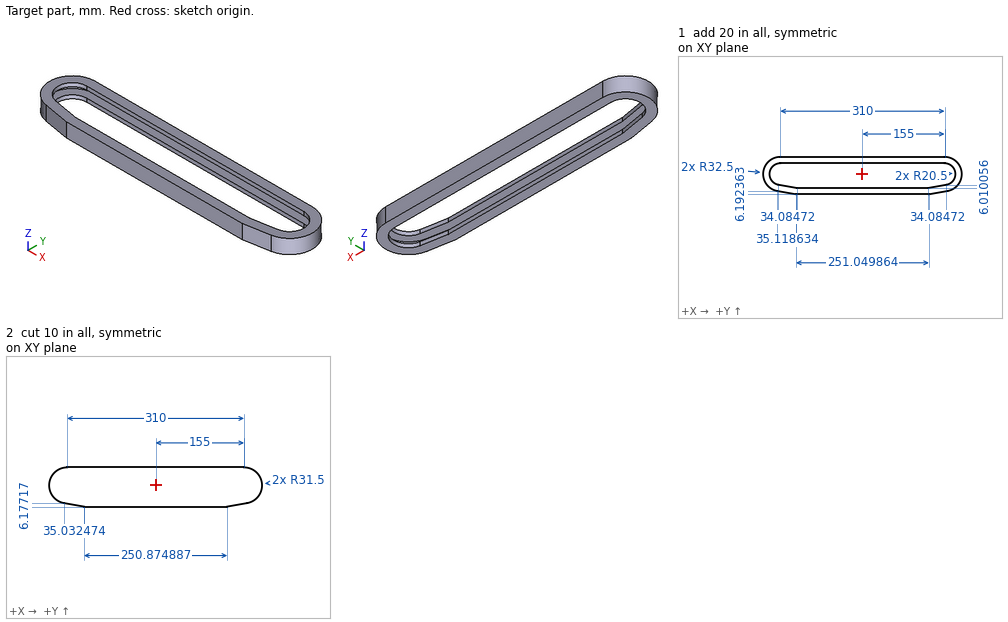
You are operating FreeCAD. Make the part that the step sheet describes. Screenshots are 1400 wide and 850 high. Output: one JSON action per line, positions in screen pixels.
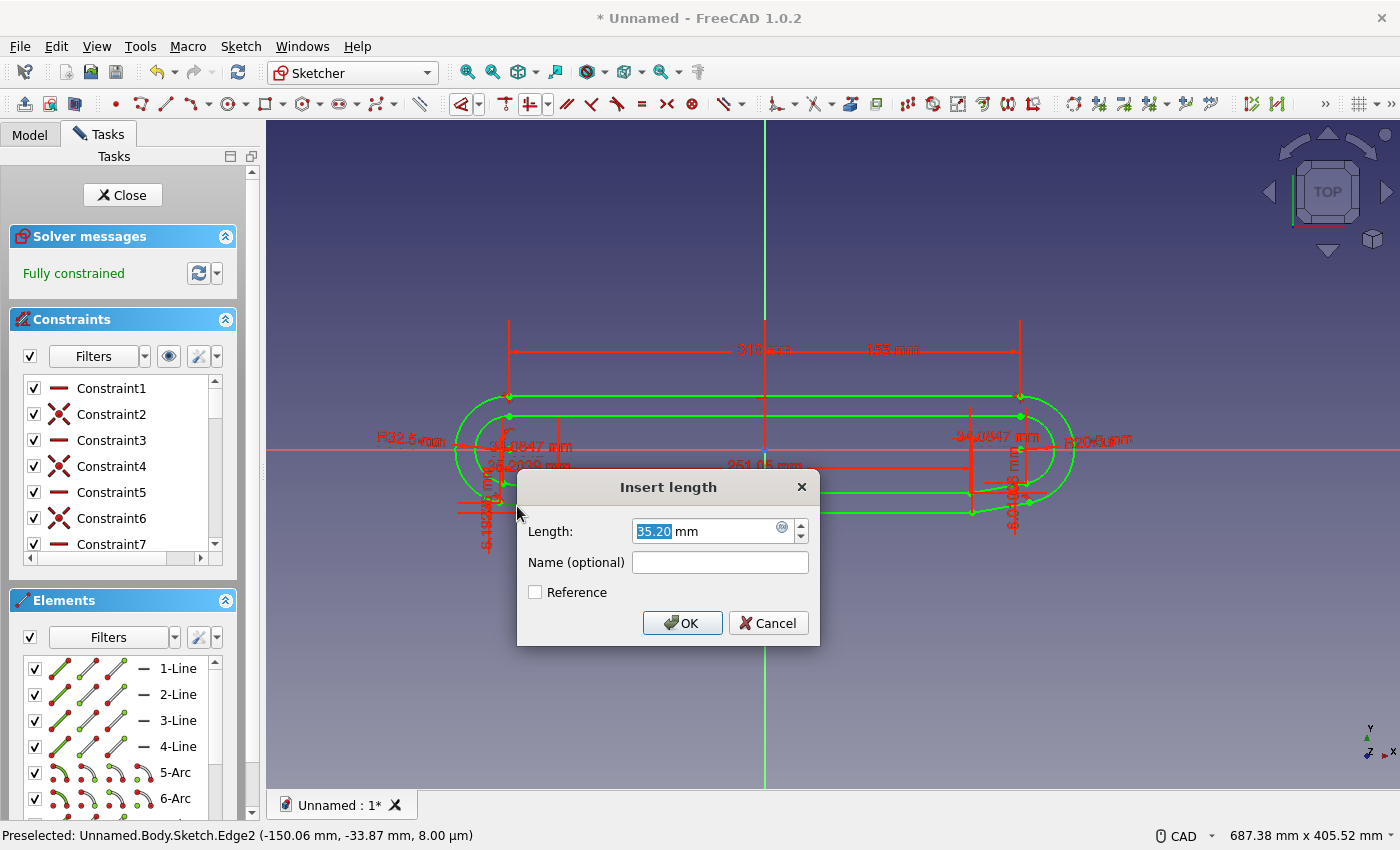
{"action": "type", "text": "35.118634"}
{"action": "key", "text": "Return"}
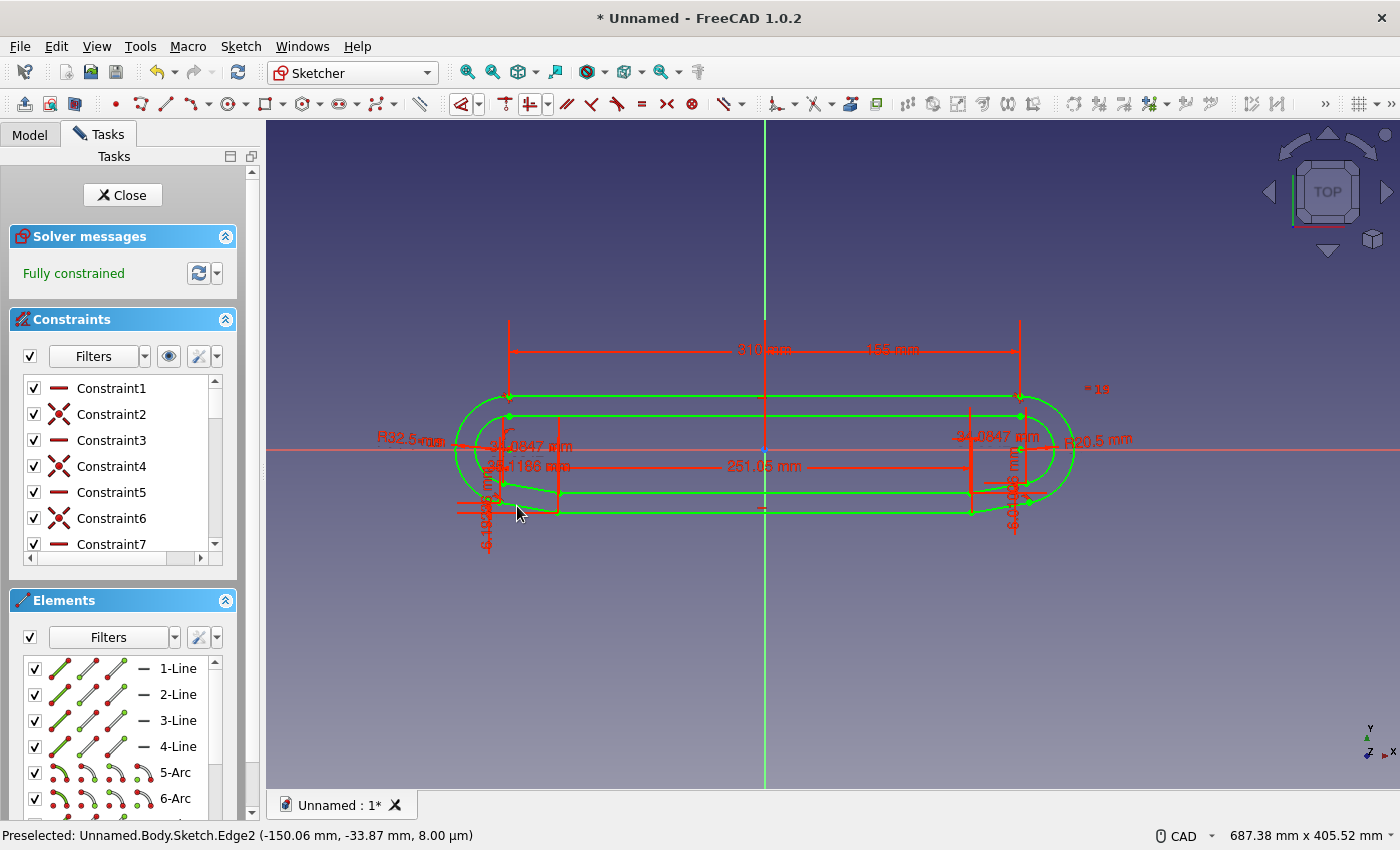
{"action": "left_click", "coordinate": [123, 195]}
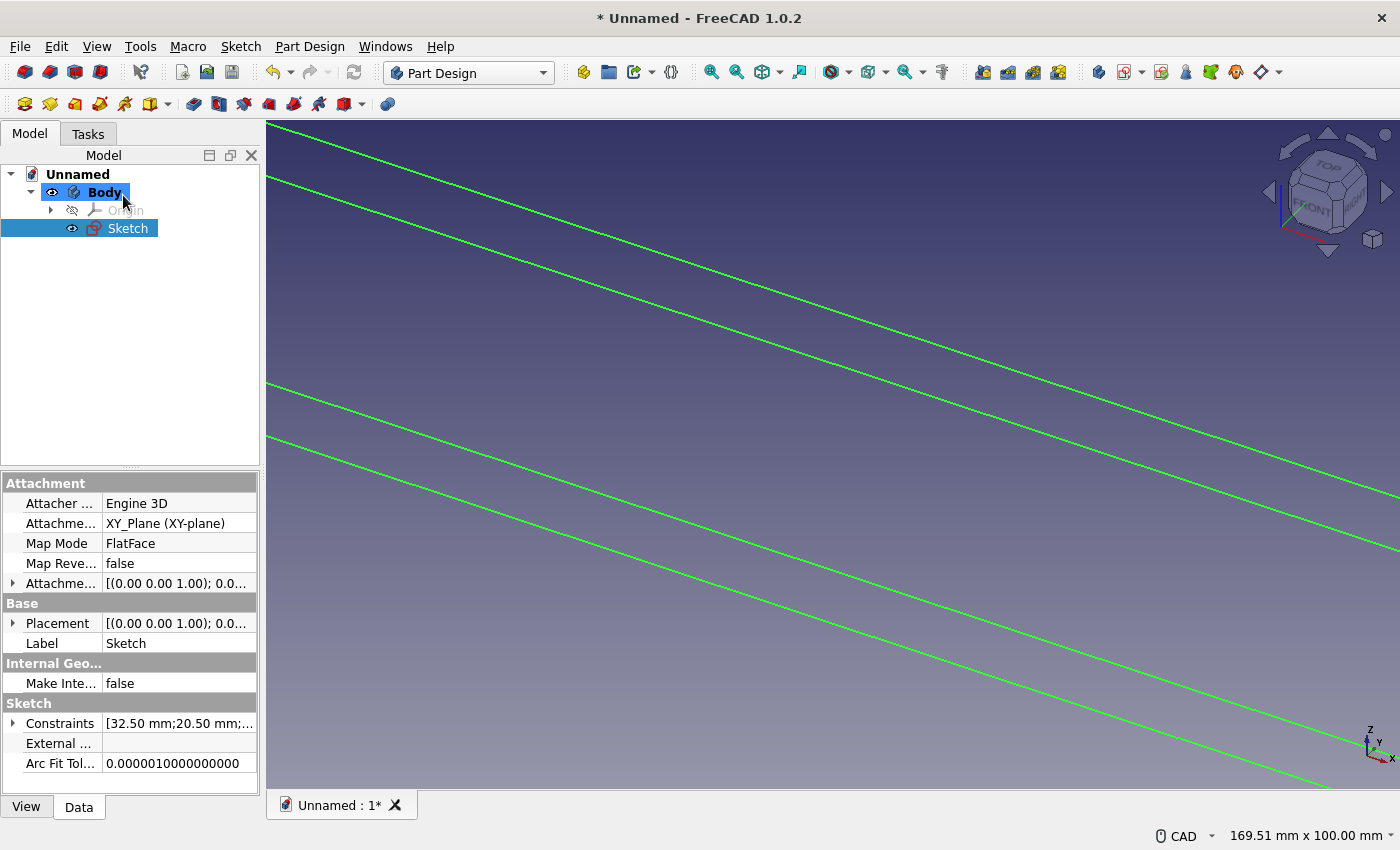
{"action": "left_click", "coordinate": [25, 104]}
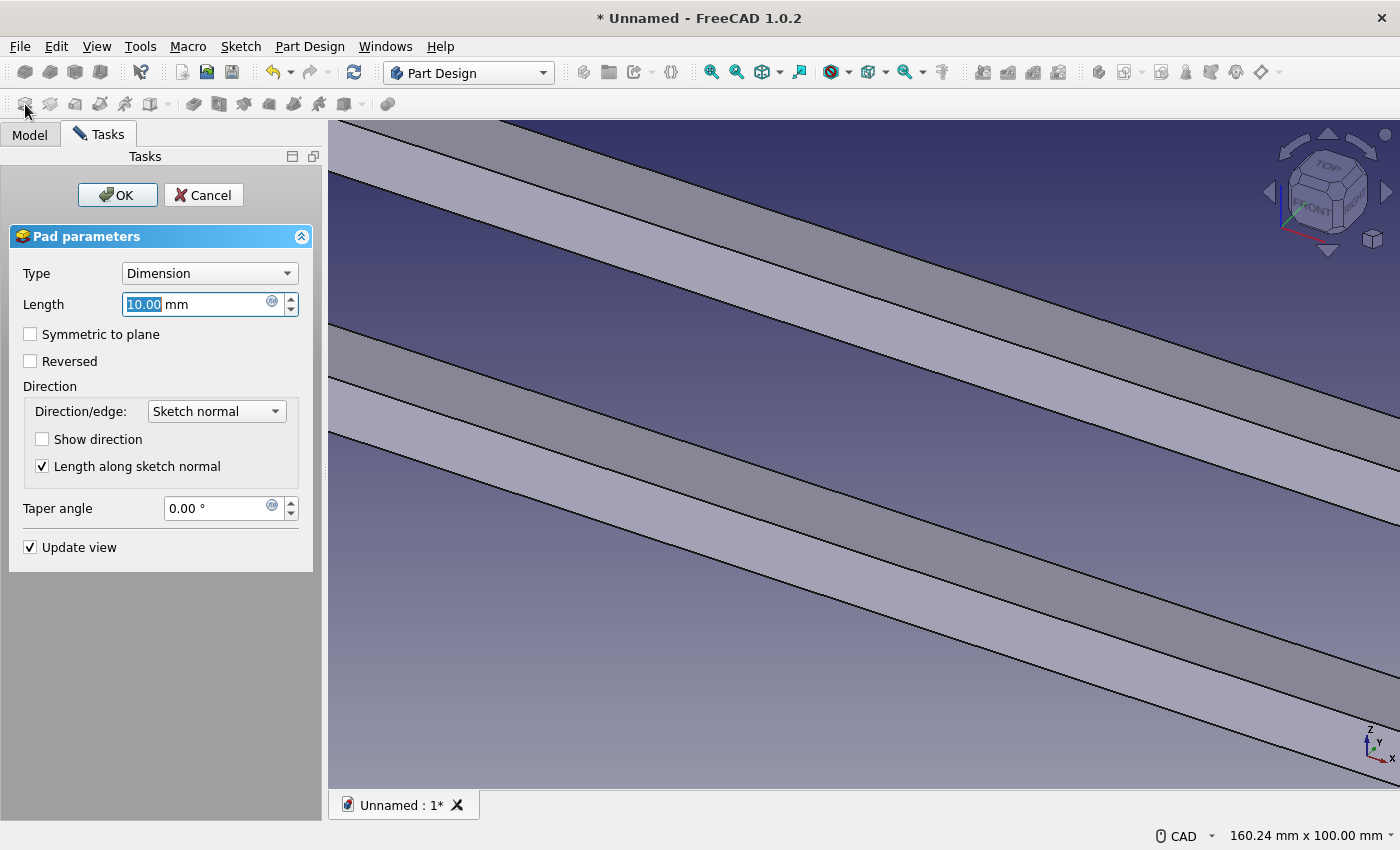
{"action": "type", "text": "20"}
{"action": "key", "text": "Tab"}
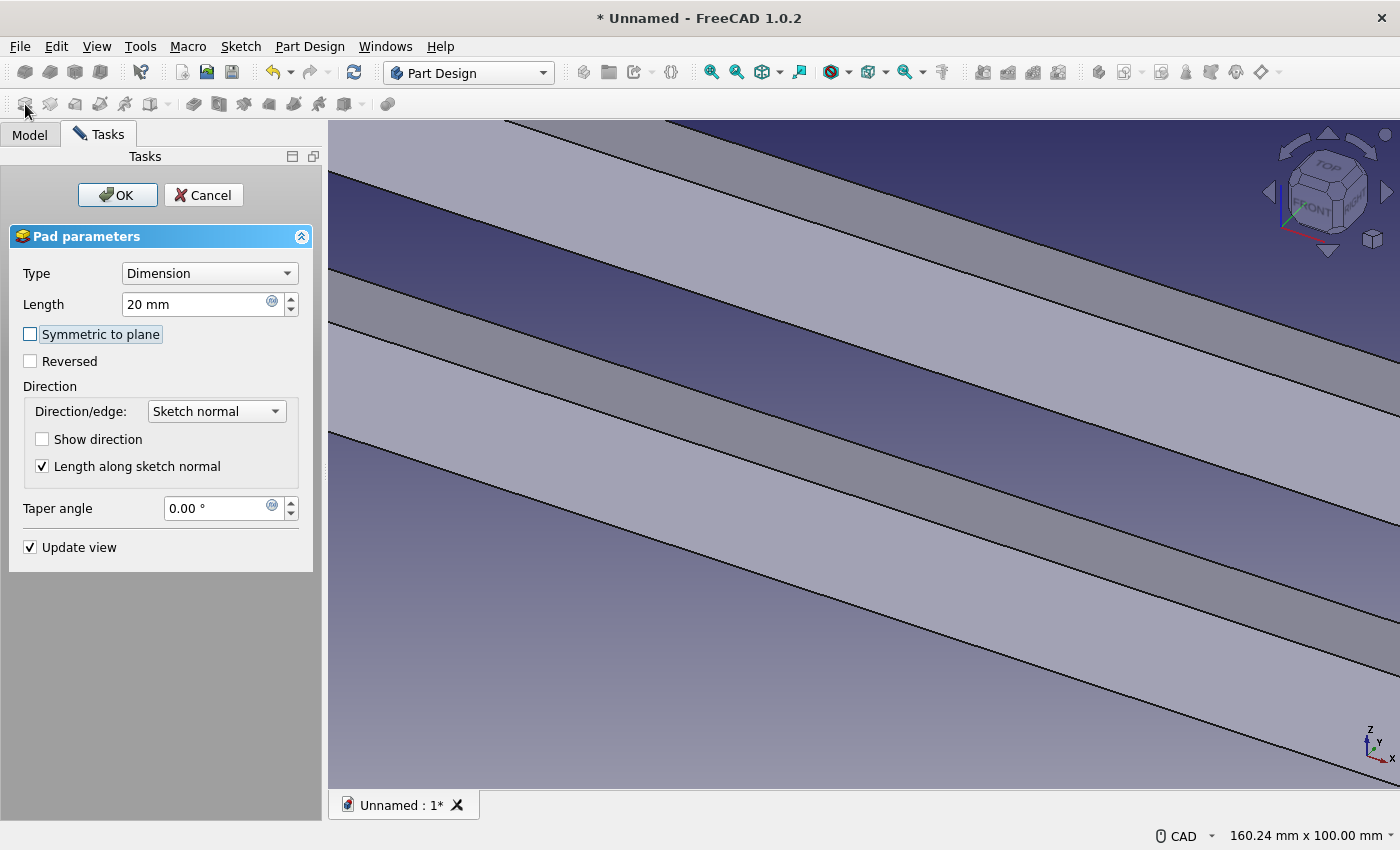
{"action": "left_click", "coordinate": [31, 334]}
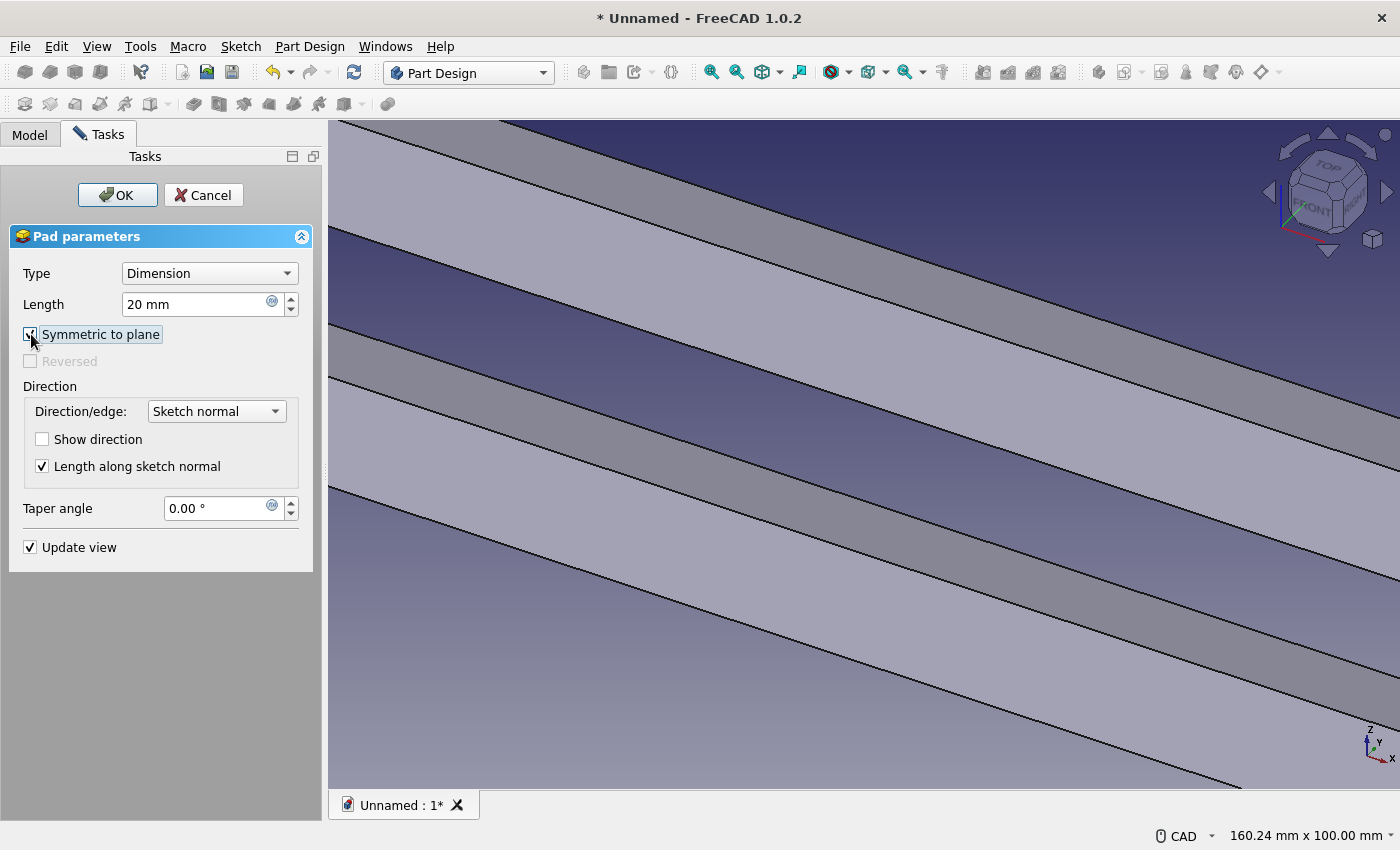
{"action": "left_click", "coordinate": [118, 195]}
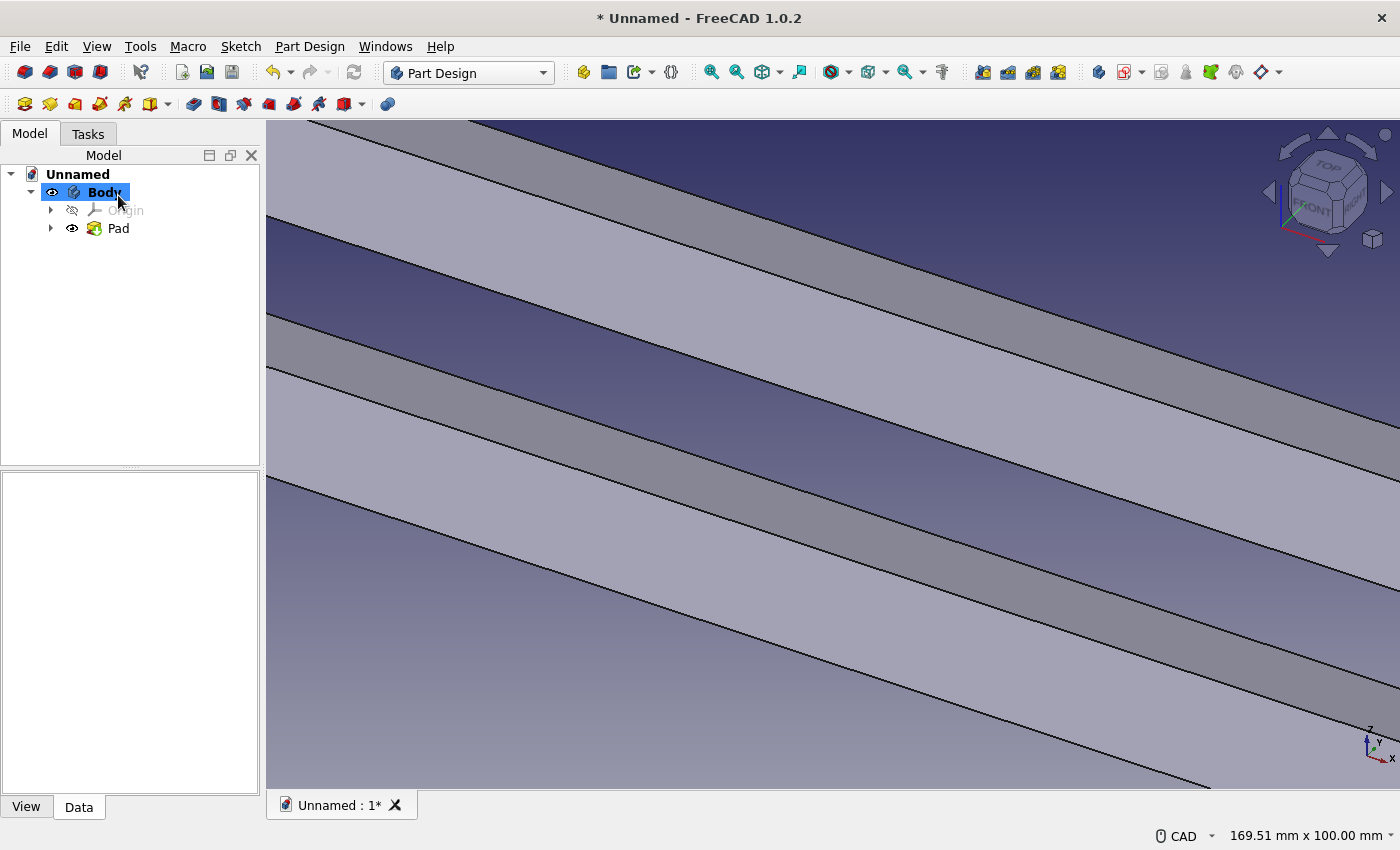
{"action": "left_click", "coordinate": [712, 72]}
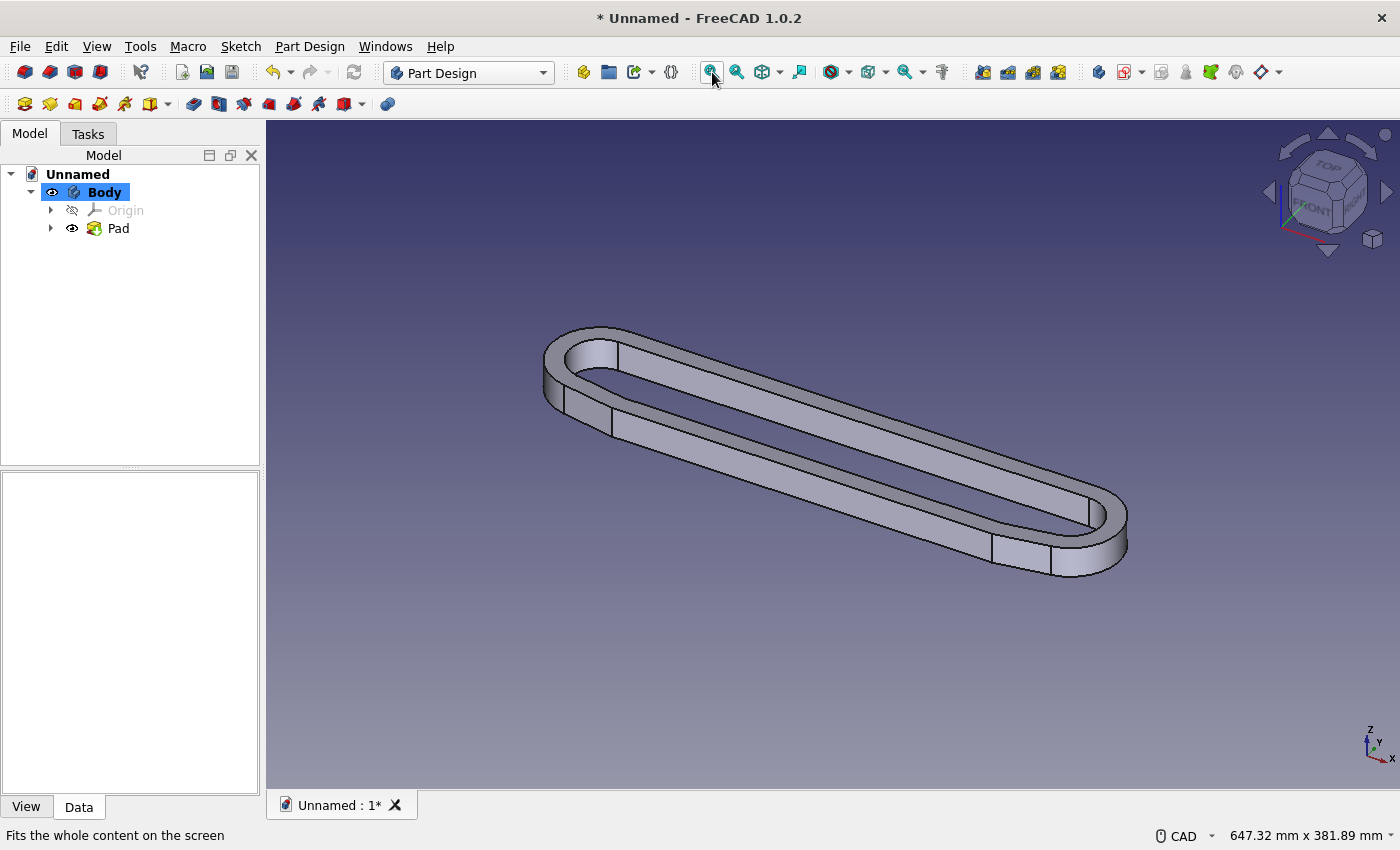
{"action": "left_click", "coordinate": [1124, 72]}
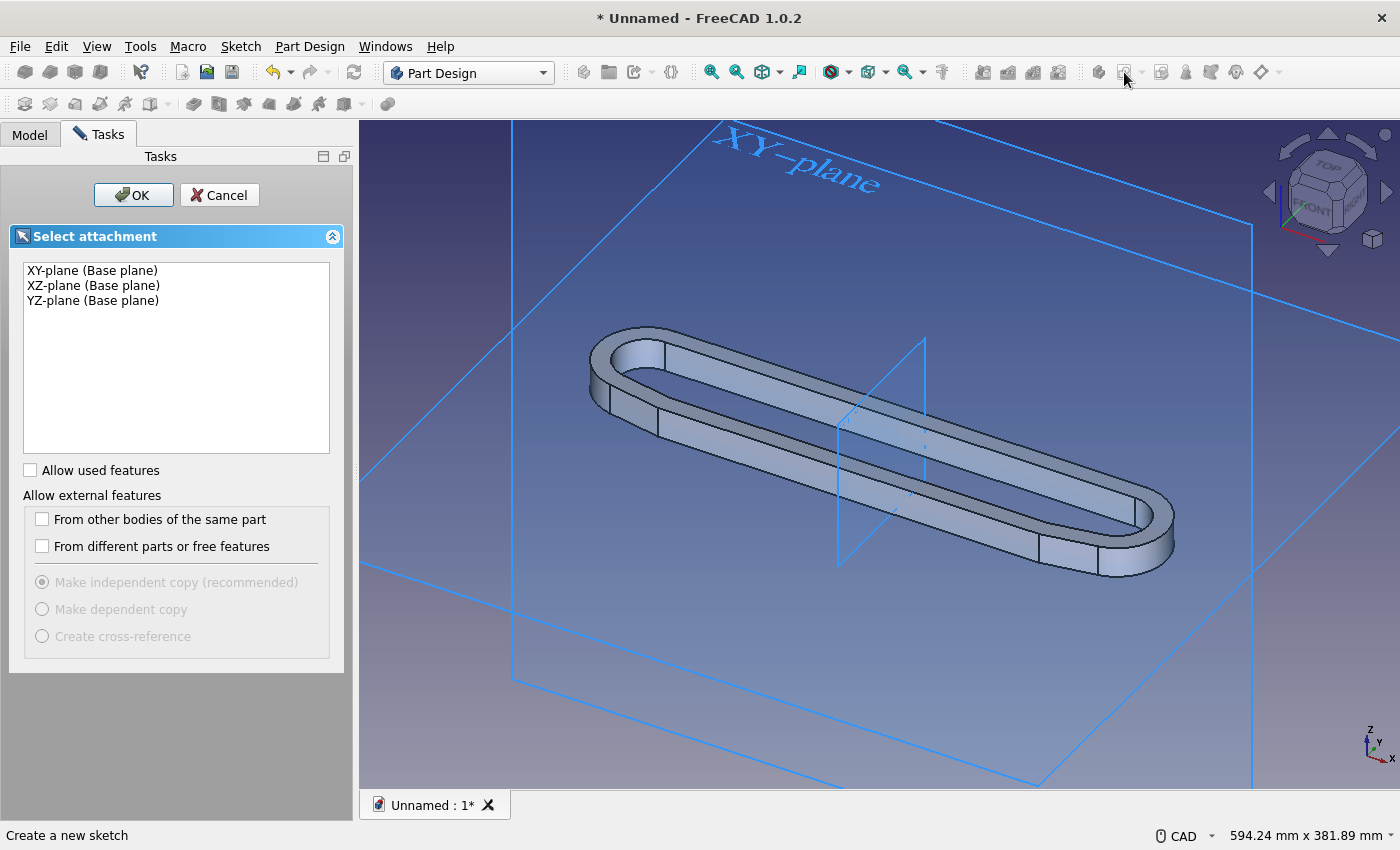
{"action": "left_click", "coordinate": [84, 270]}